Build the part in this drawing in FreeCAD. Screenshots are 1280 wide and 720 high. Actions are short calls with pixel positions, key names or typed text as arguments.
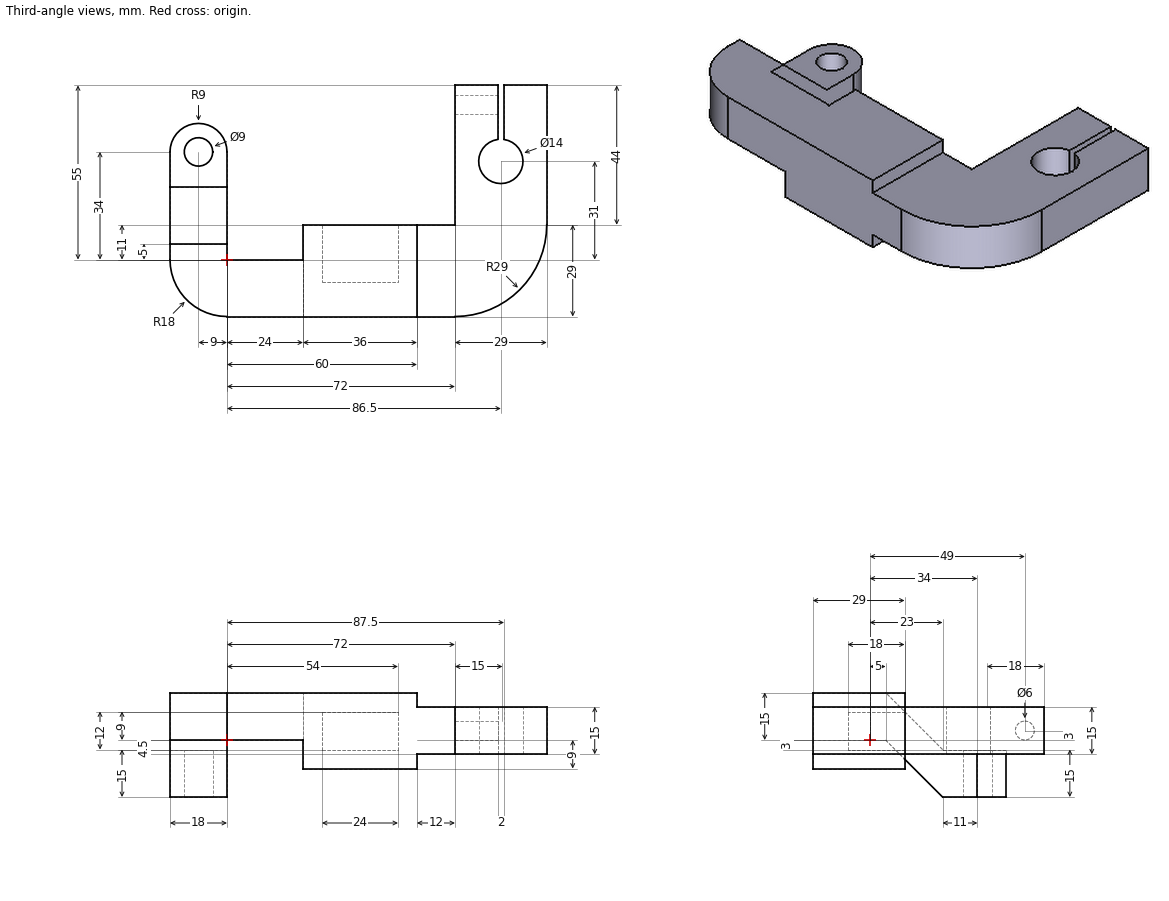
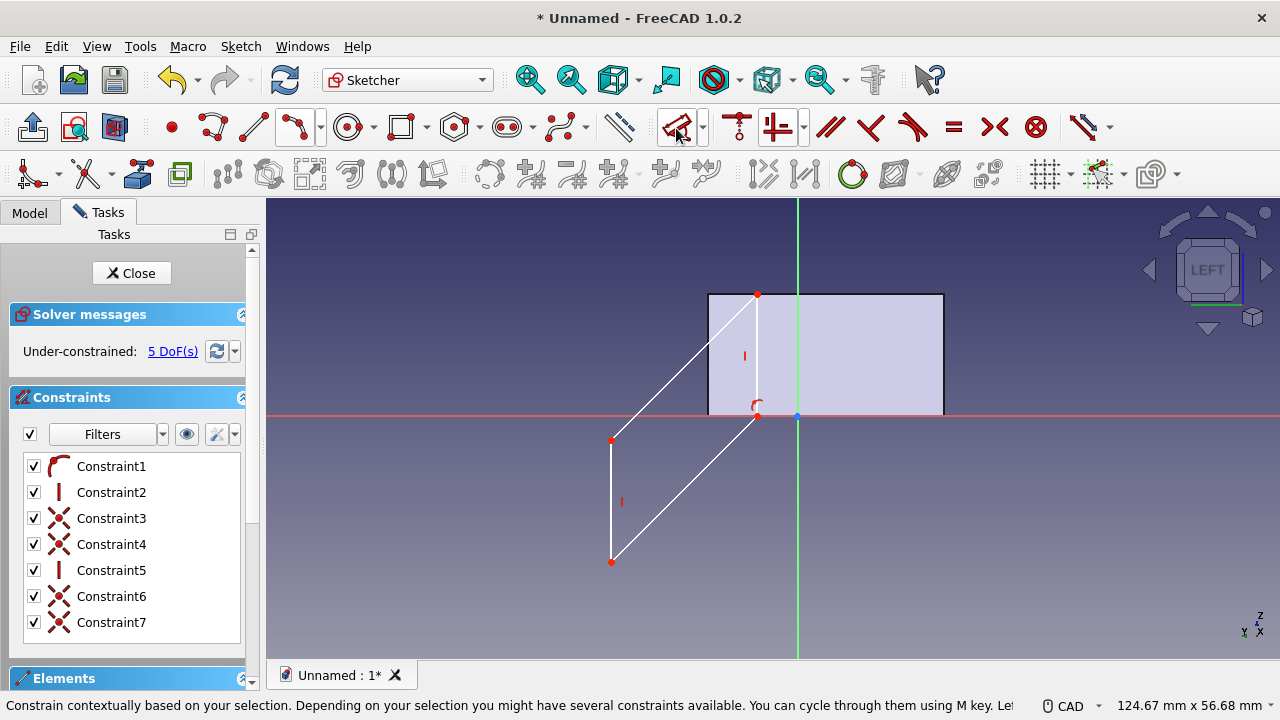
click(757, 380)
click(723, 356)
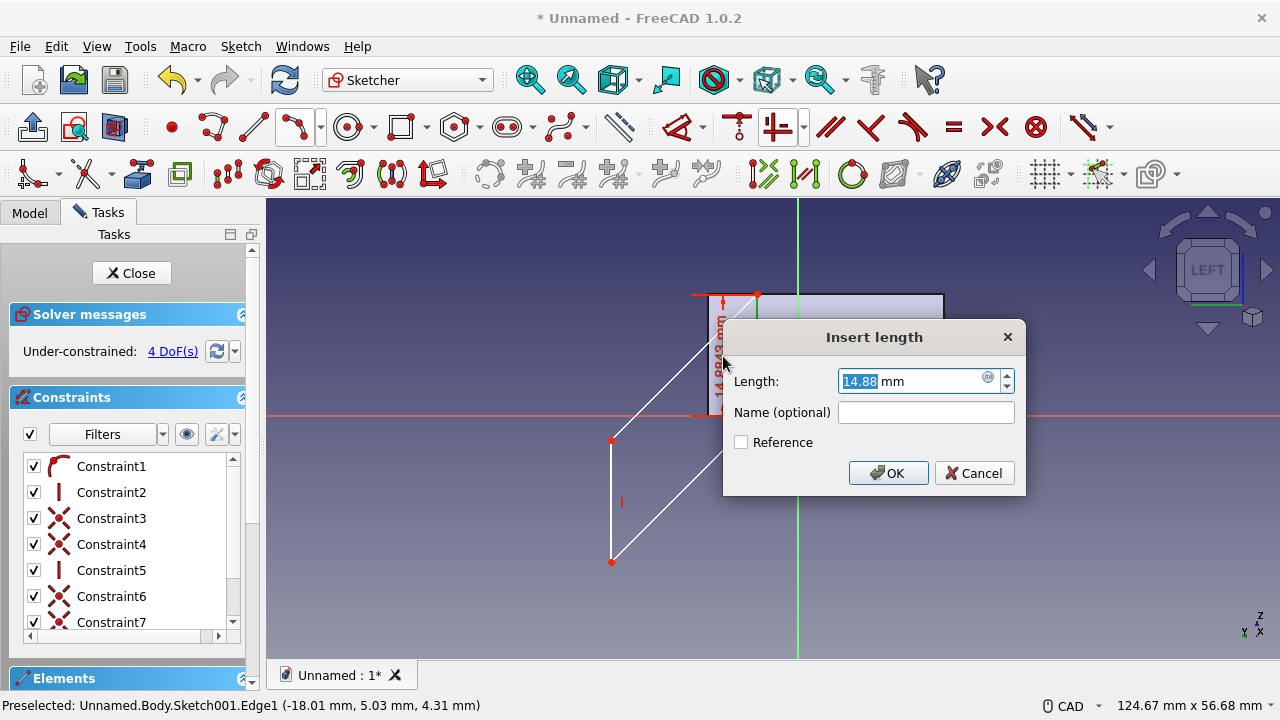
text(15)
key(Return)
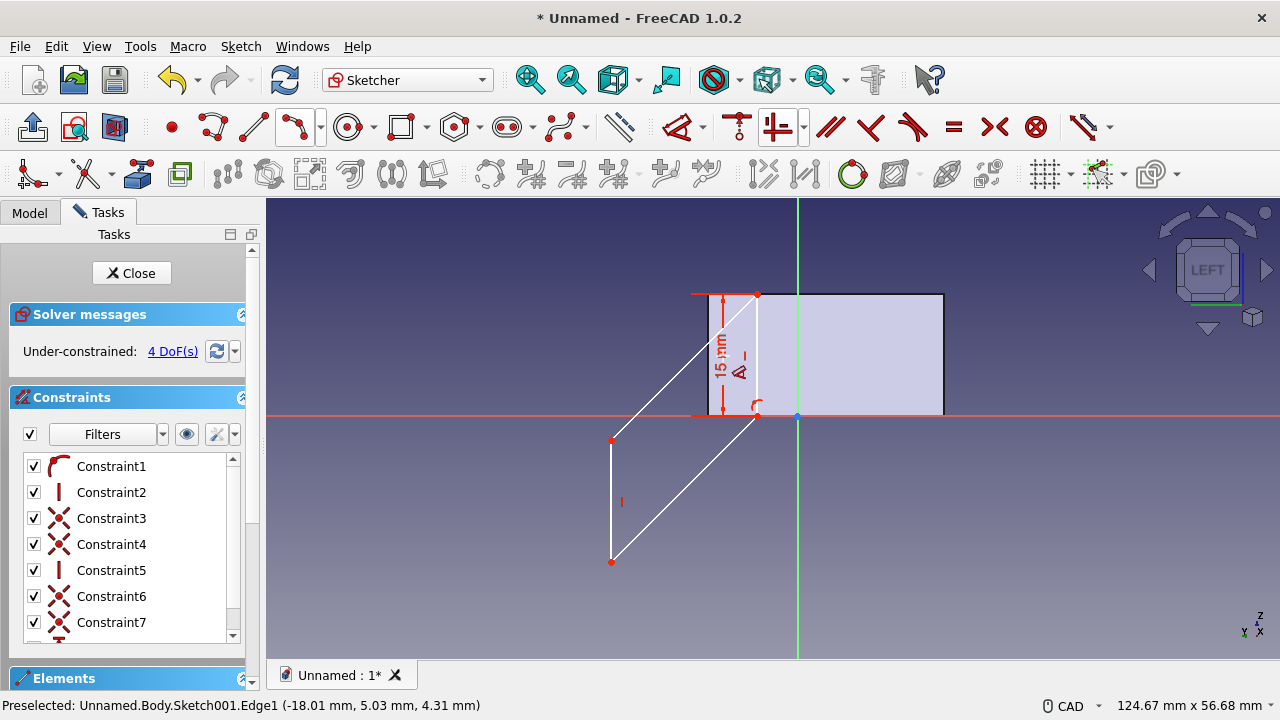
click(611, 478)
click(577, 502)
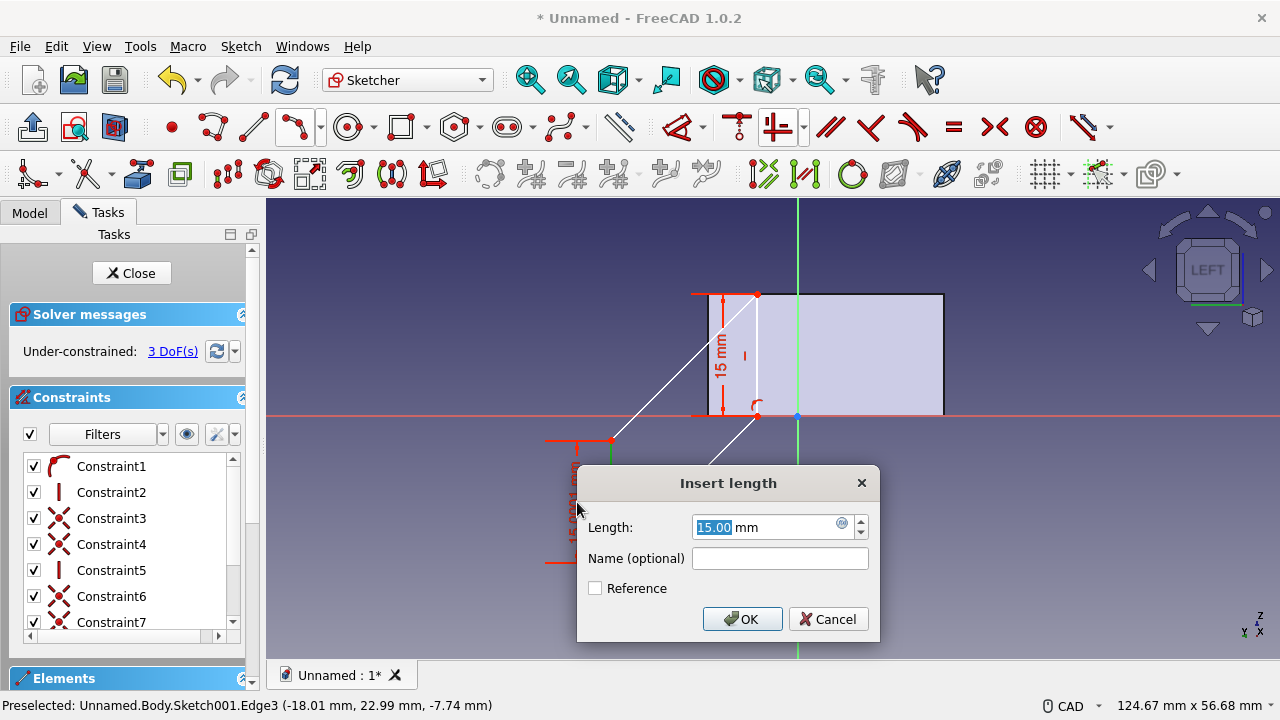
text(15)
key(Return)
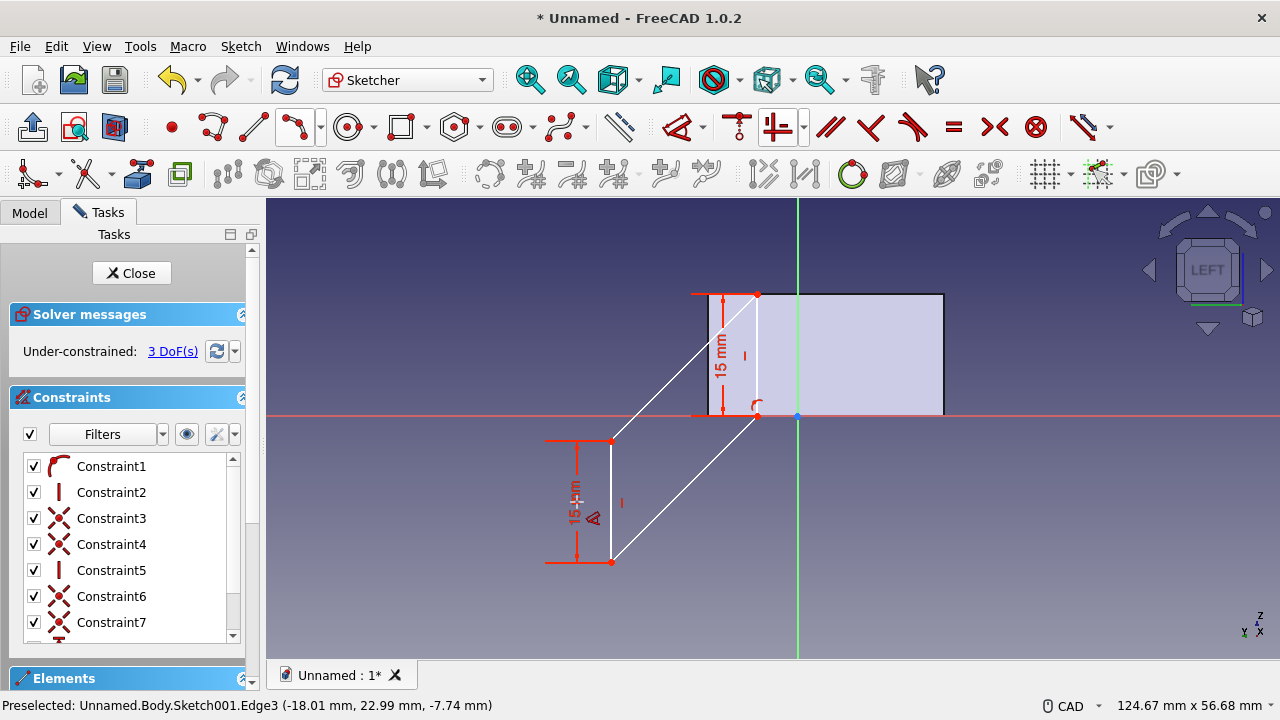
click(757, 416)
click(777, 382)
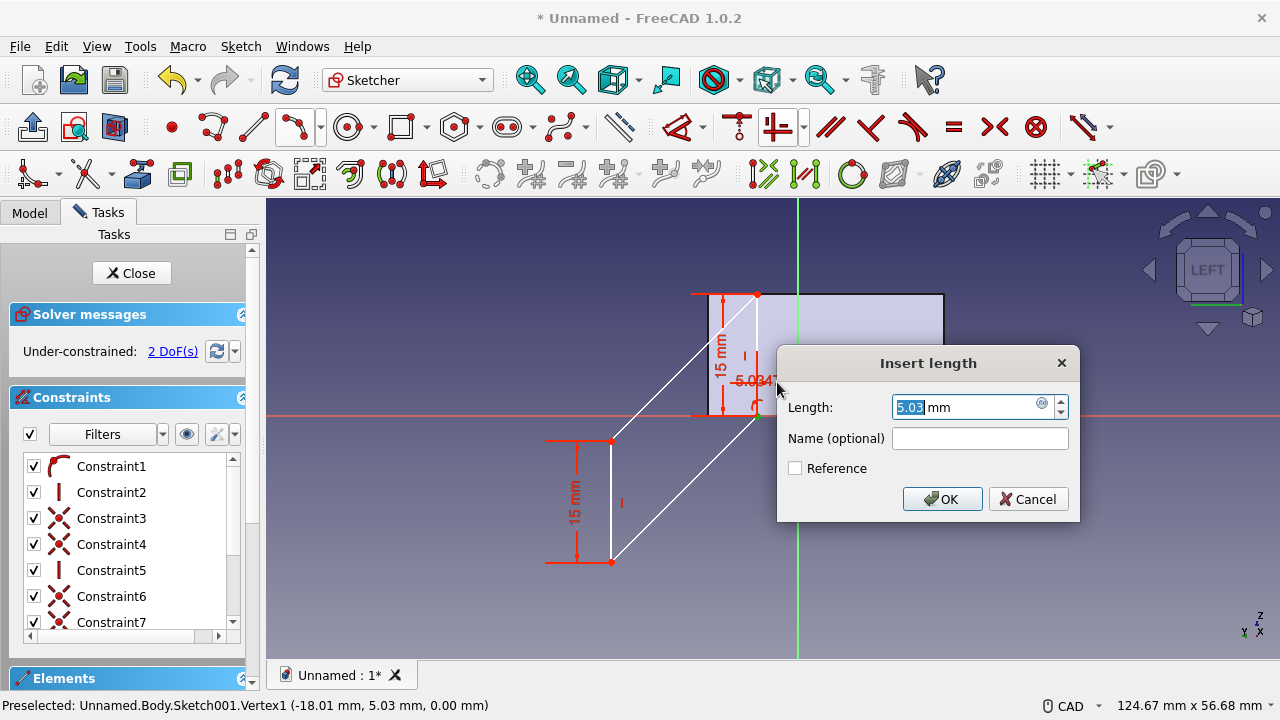
text(5)
key(Return)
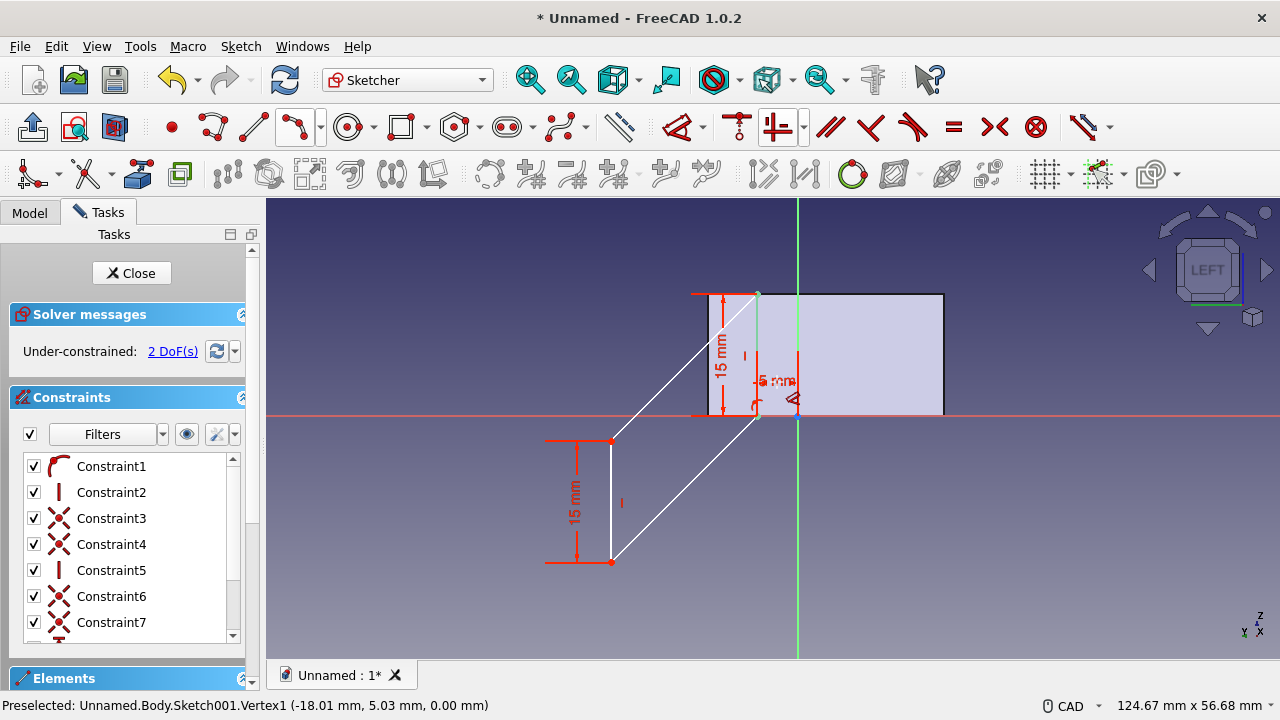
scroll(611, 441, up, 3)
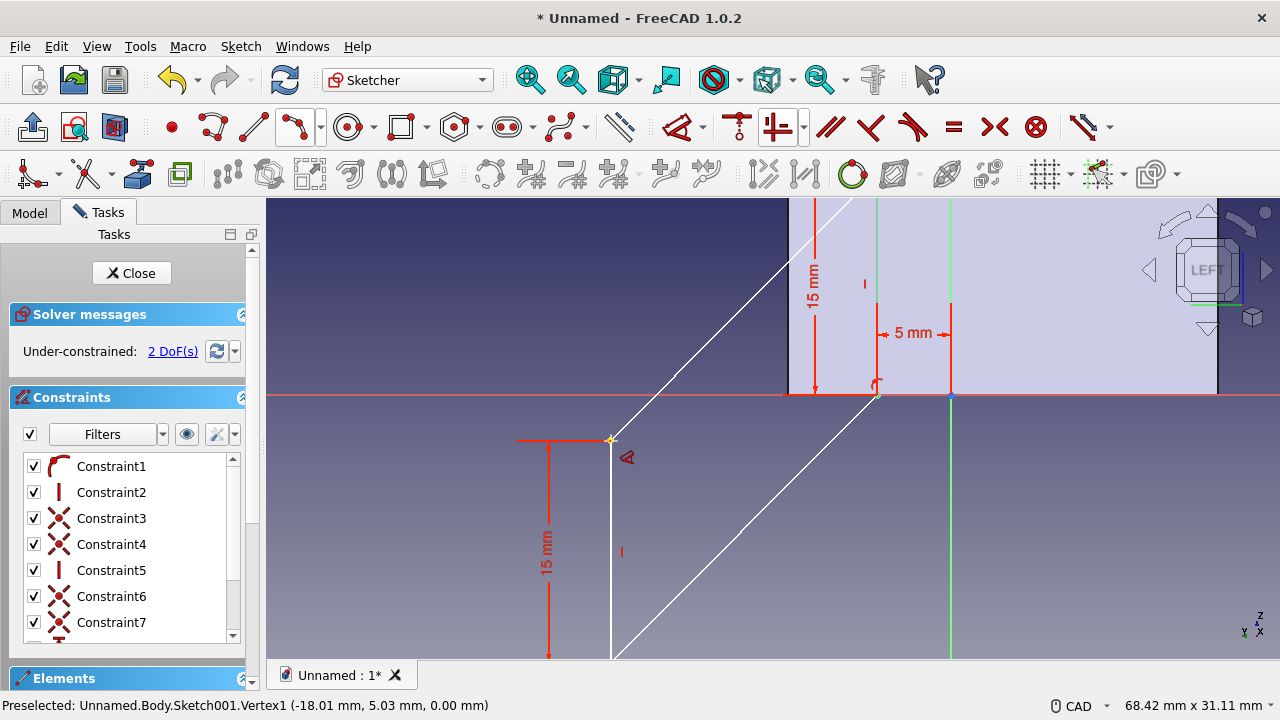
click(611, 441)
click(985, 418)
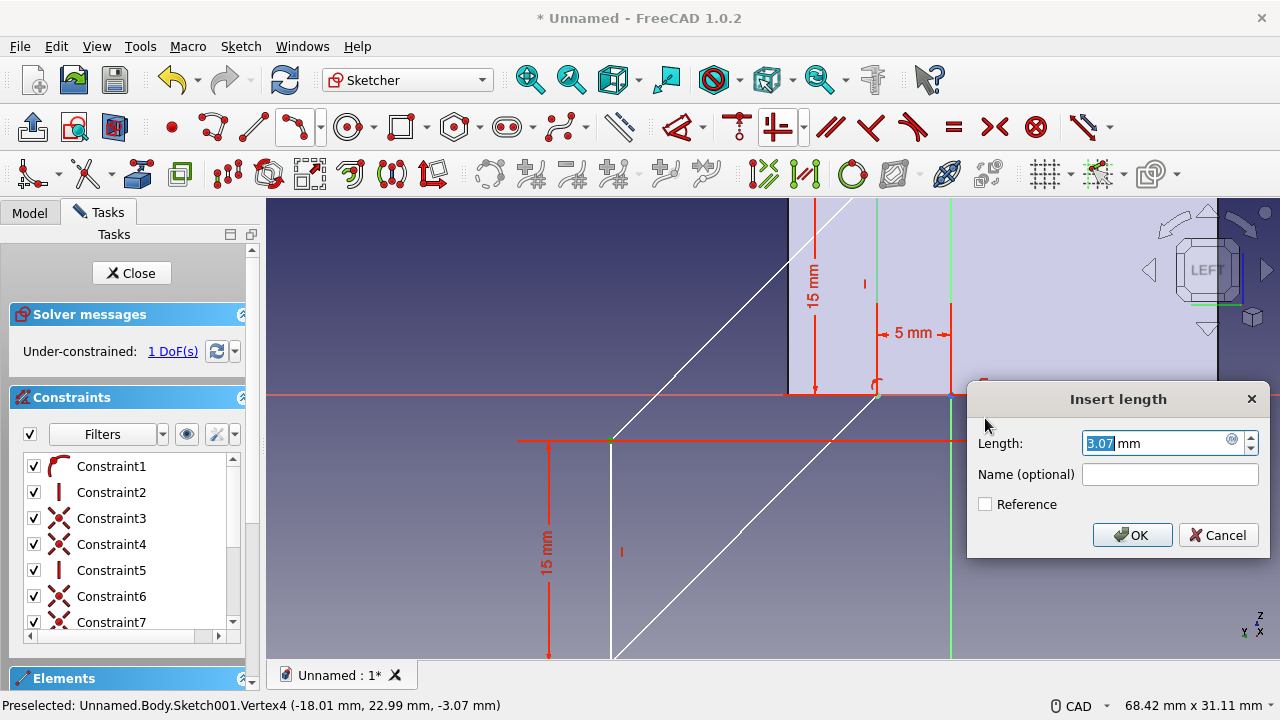
text(3)
key(Return)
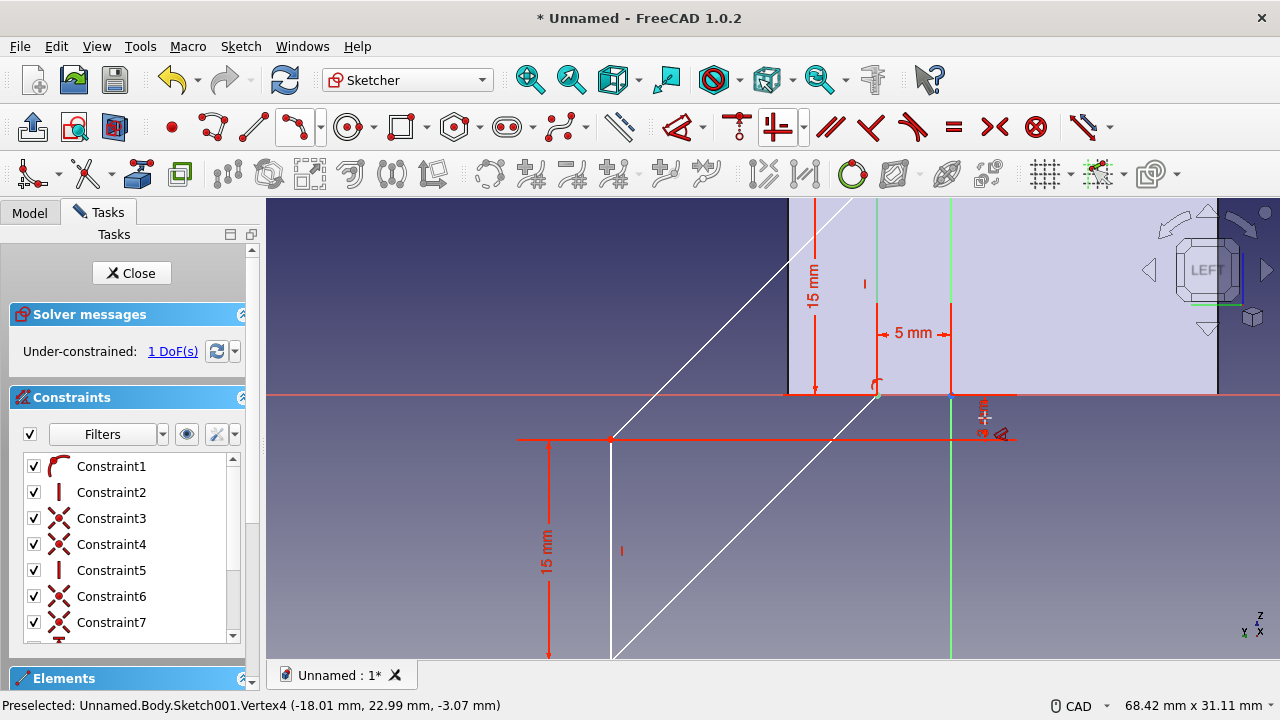
click(611, 440)
click(781, 361)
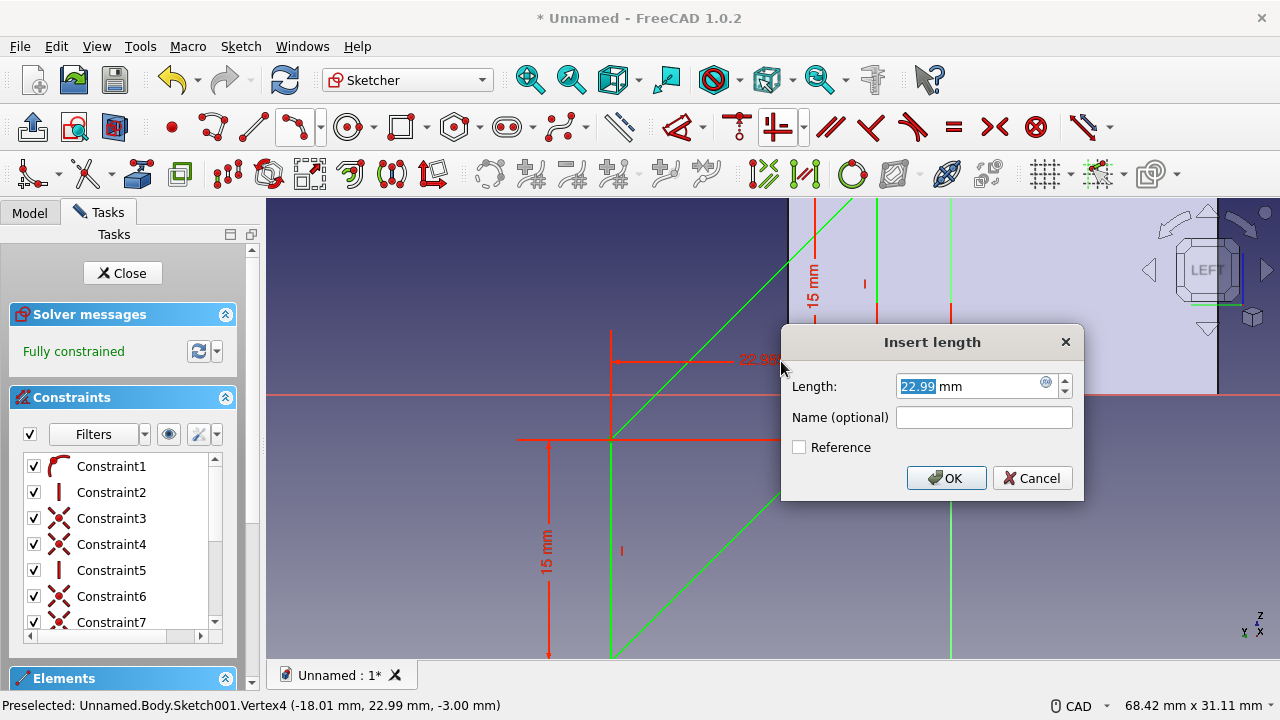
text(23)
key(Return)
key(Escape)